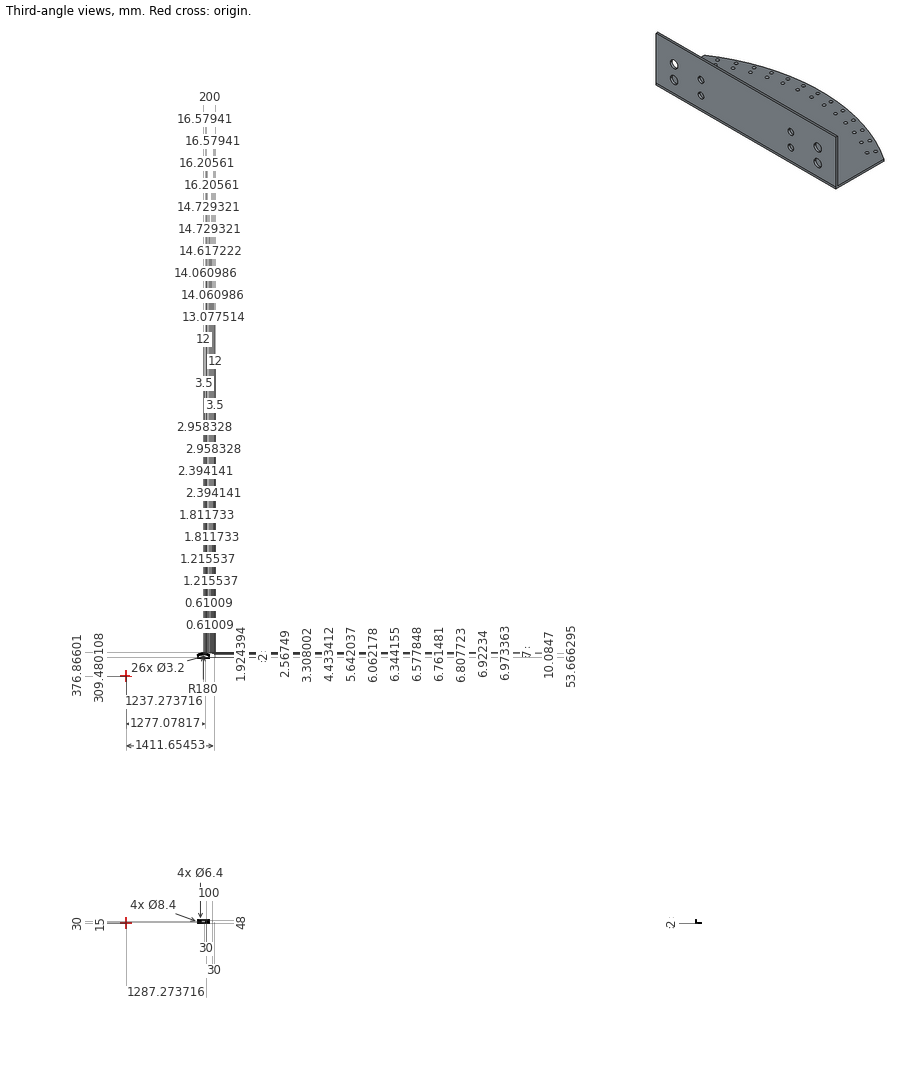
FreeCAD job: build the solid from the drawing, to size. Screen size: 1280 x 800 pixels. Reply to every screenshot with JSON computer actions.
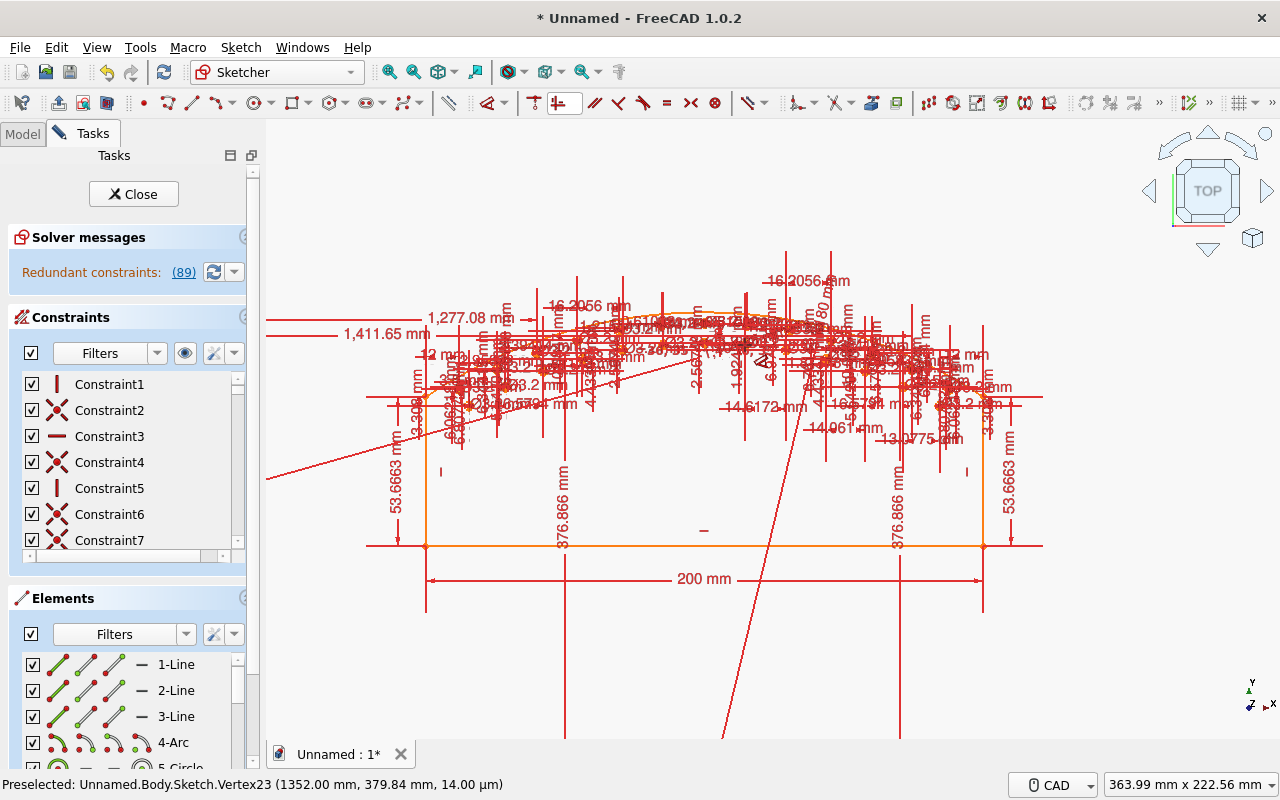
{"action": "left_click", "coordinate": [705, 343]}
{"action": "left_click", "coordinate": [725, 379]}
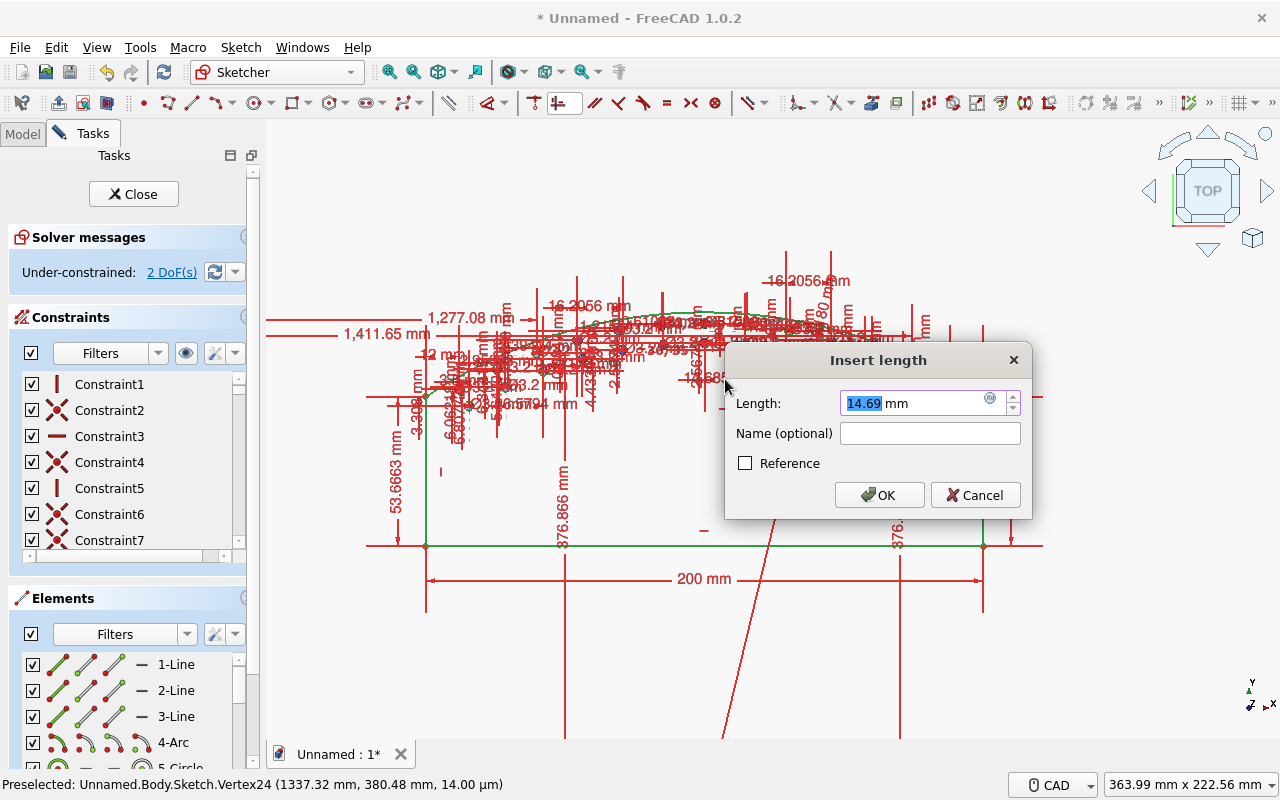
{"action": "type", "text": "14.729321"}
{"action": "key", "text": "Return"}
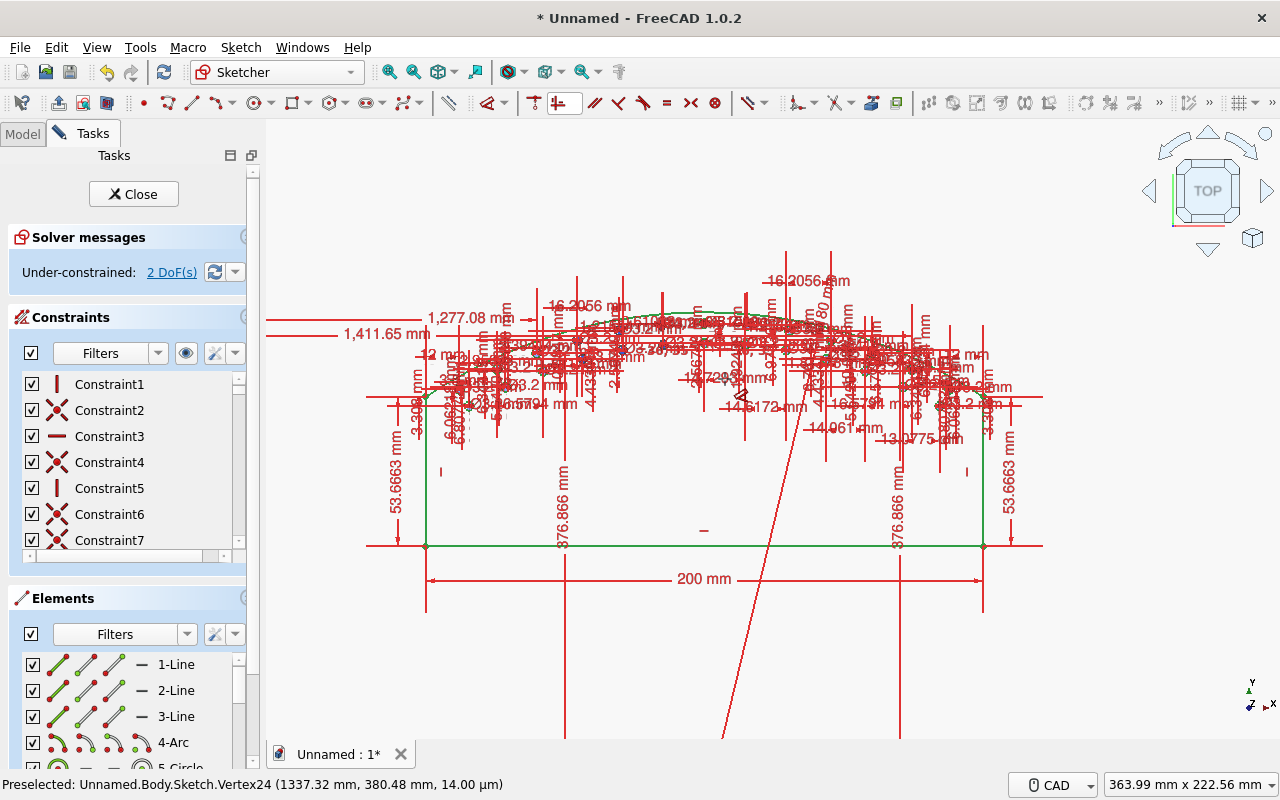
{"action": "left_click", "coordinate": [543, 371]}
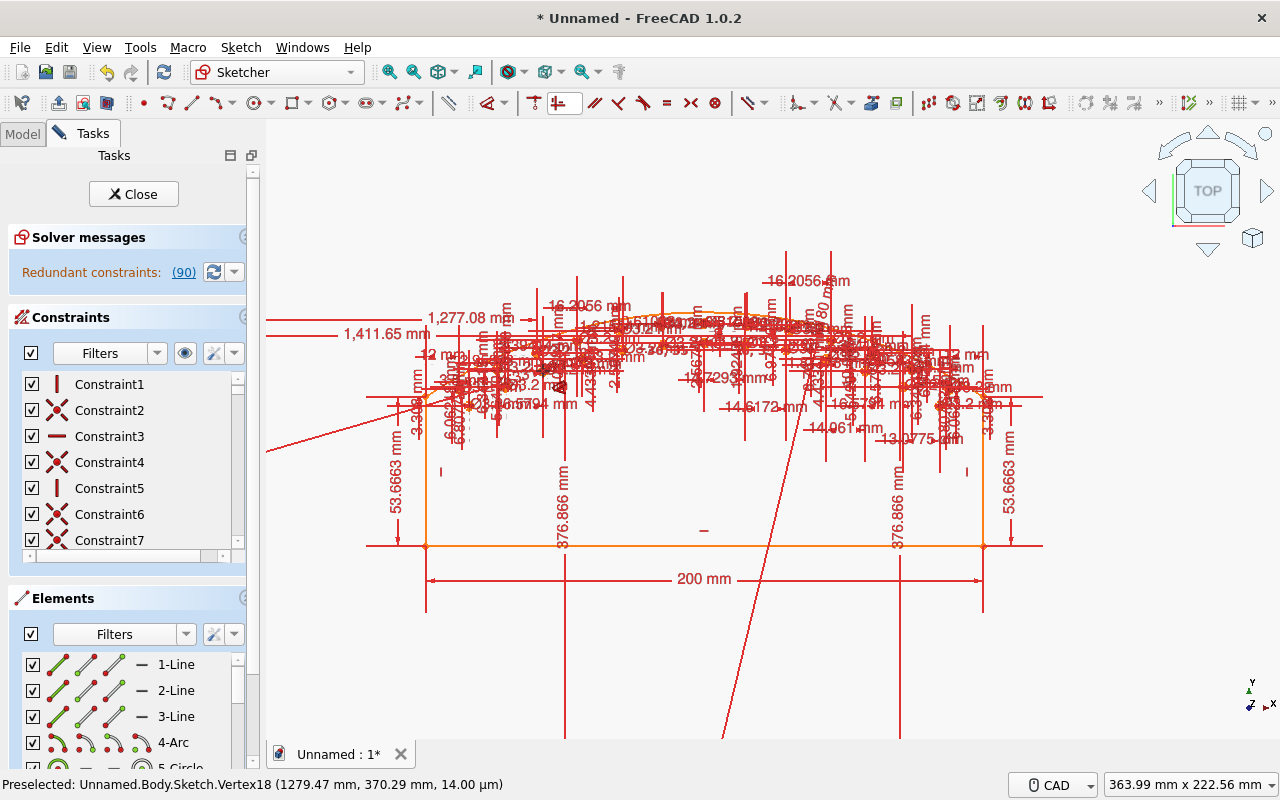
{"action": "left_click", "coordinate": [583, 359]}
{"action": "left_click", "coordinate": [563, 429]}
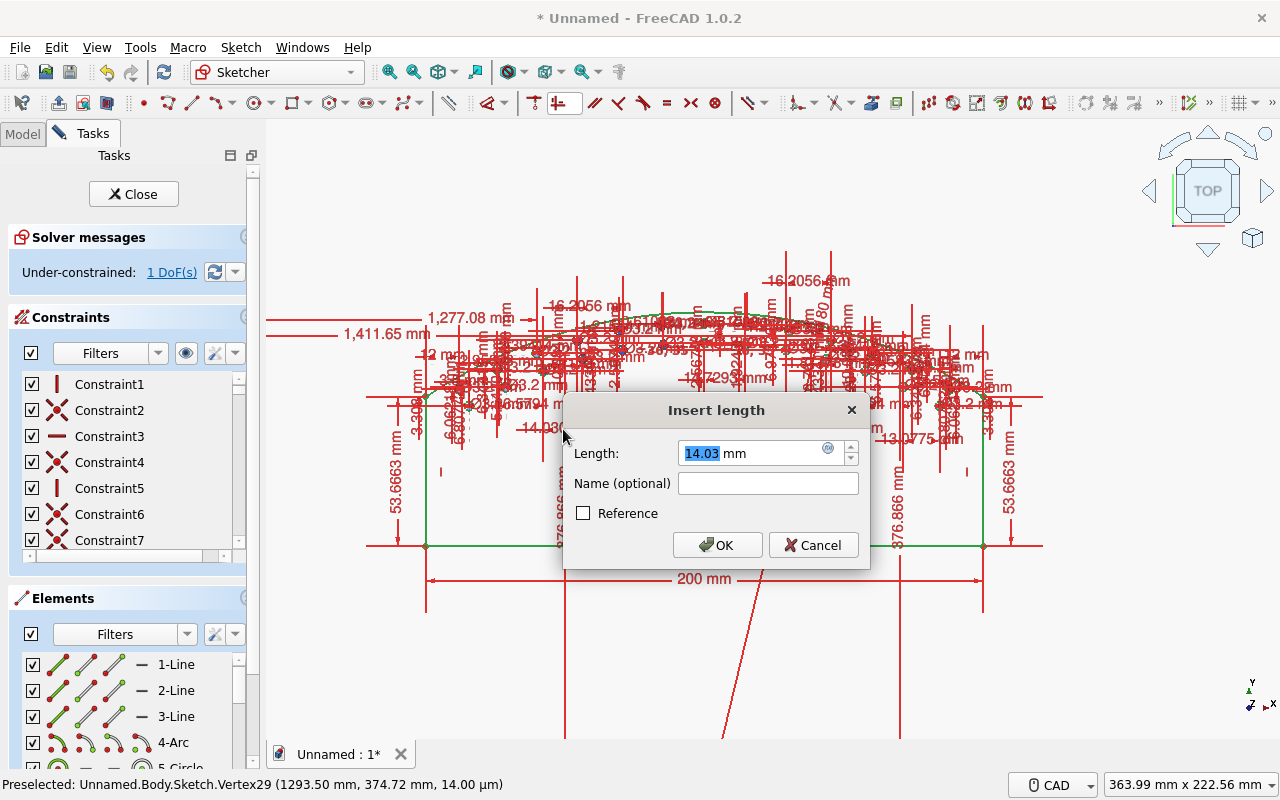
{"action": "type", "text": "14.060986"}
{"action": "key", "text": "Return"}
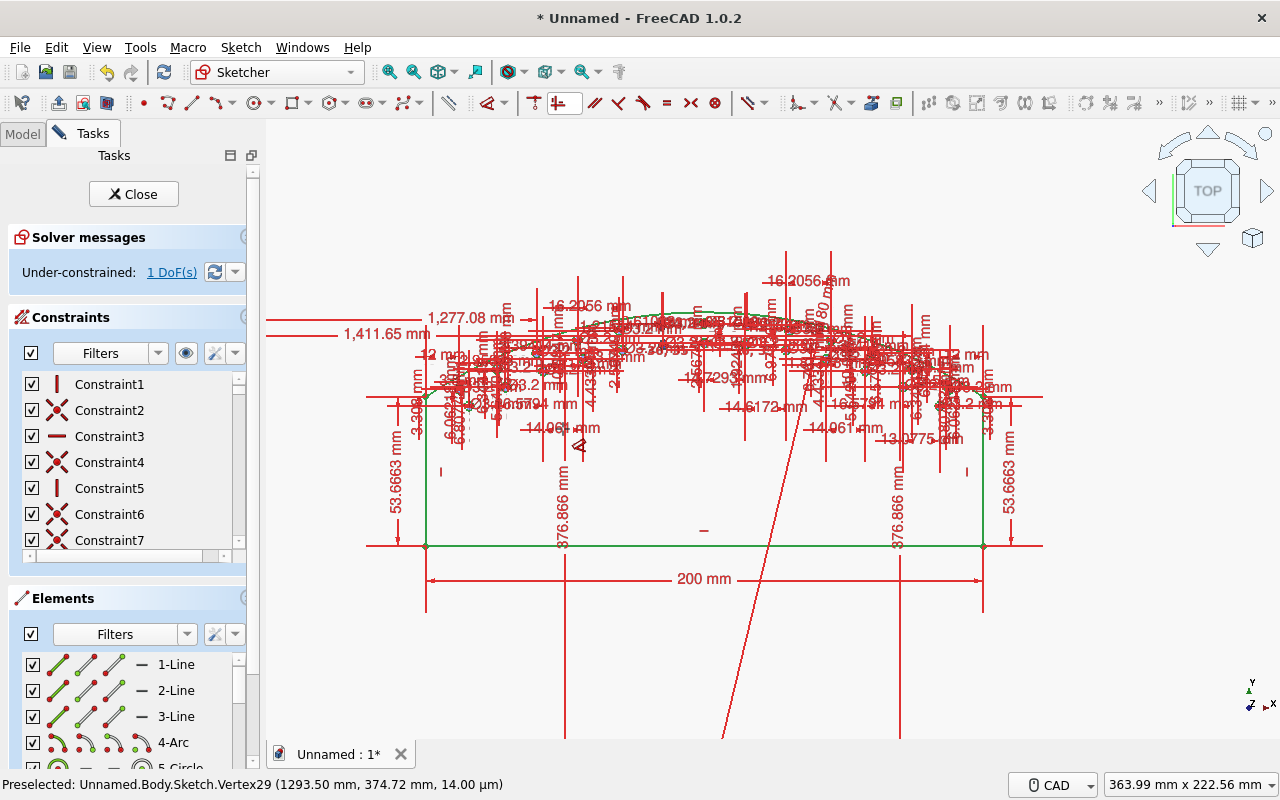
{"action": "left_click", "coordinate": [704, 343]}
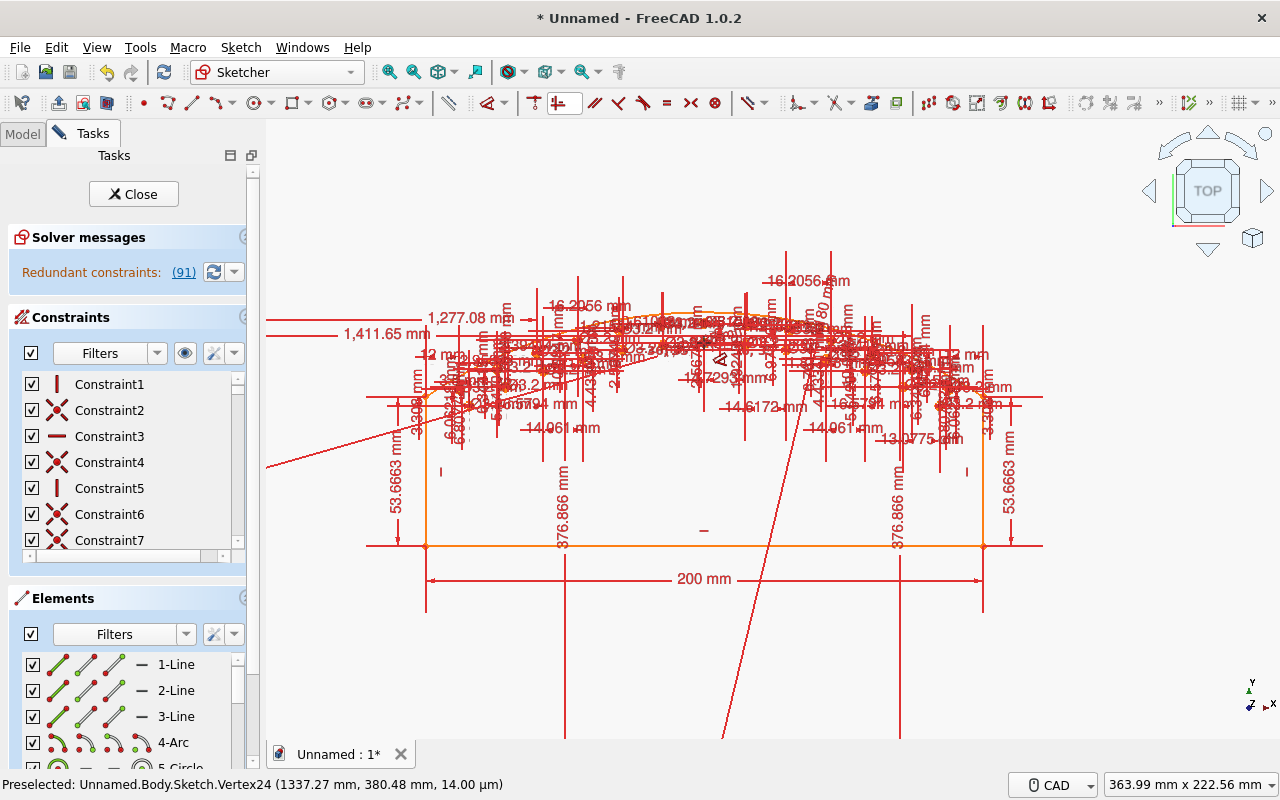
{"action": "left_click", "coordinate": [663, 345]}
{"action": "left_click", "coordinate": [684, 285]}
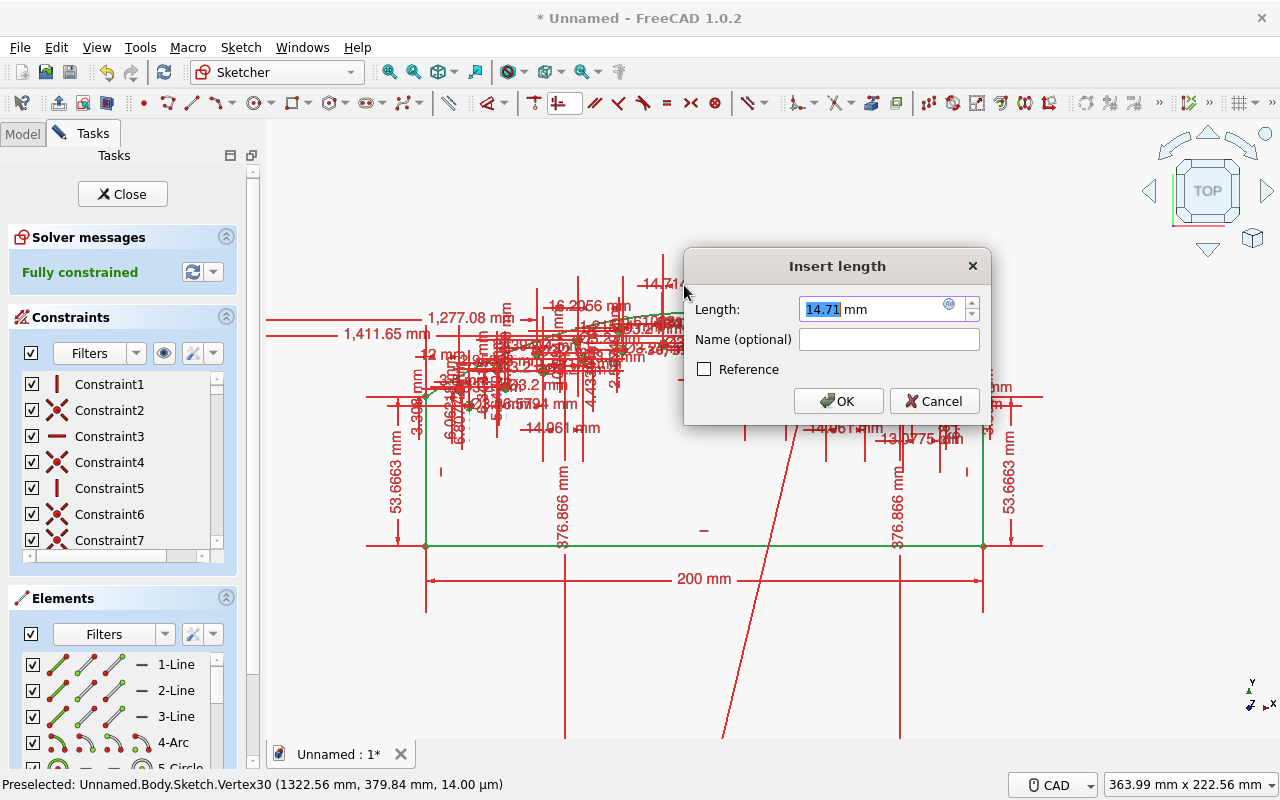
{"action": "type", "text": "14.729321"}
{"action": "key", "text": "Return"}
{"action": "key", "text": "Escape"}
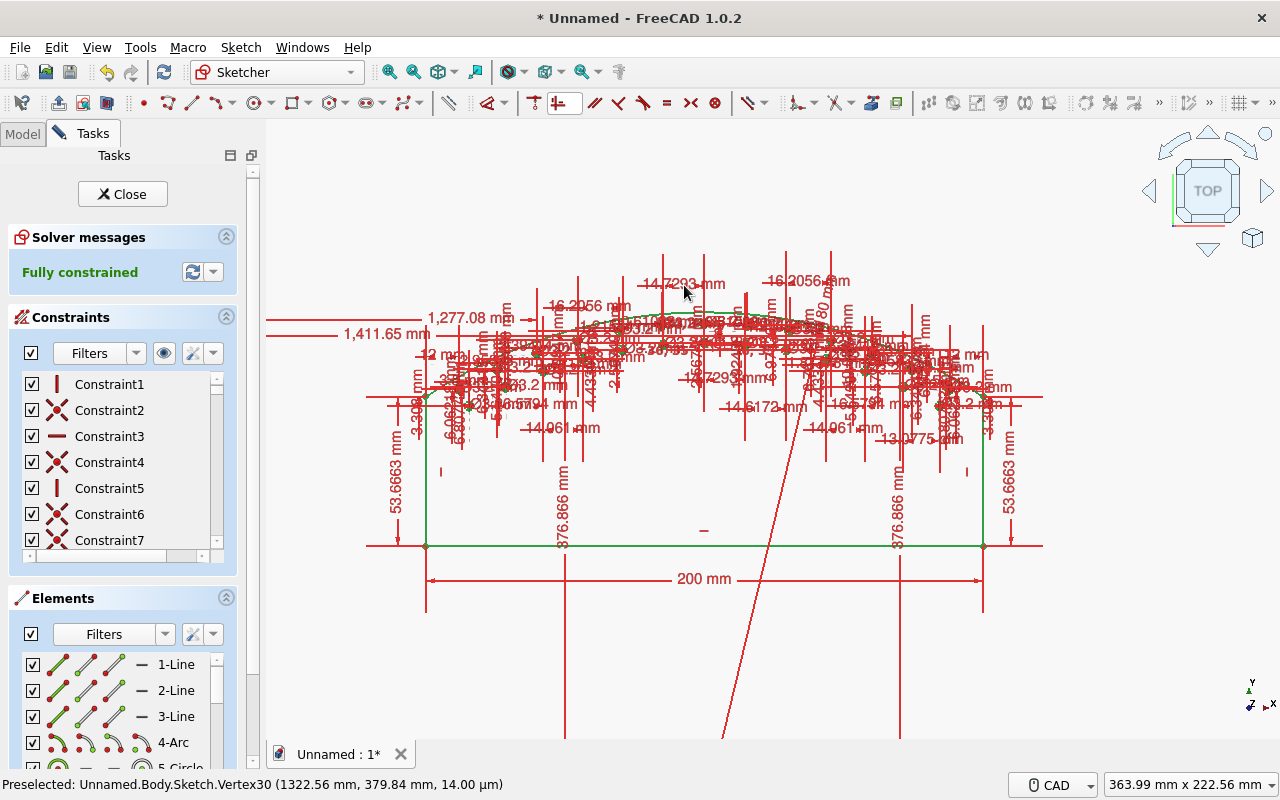
{"action": "left_click", "coordinate": [123, 194]}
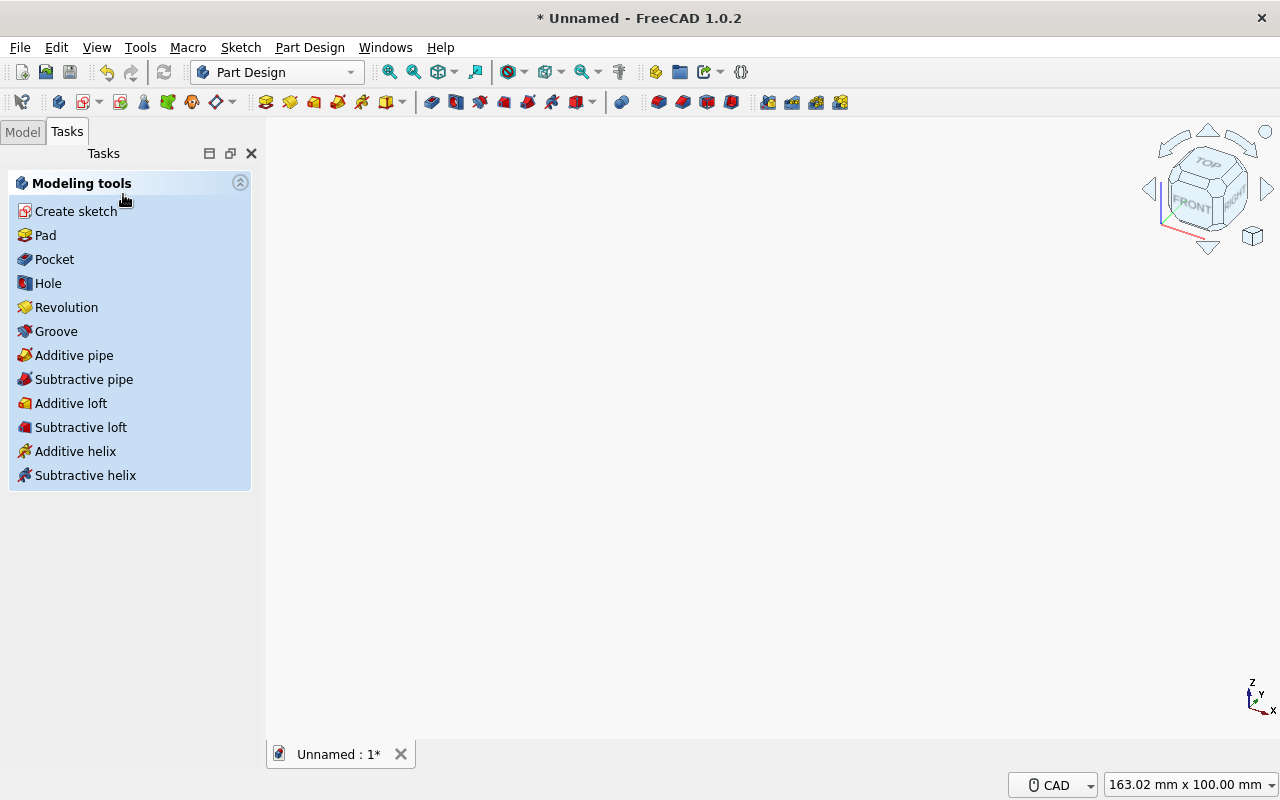
{"action": "left_click", "coordinate": [266, 102]}